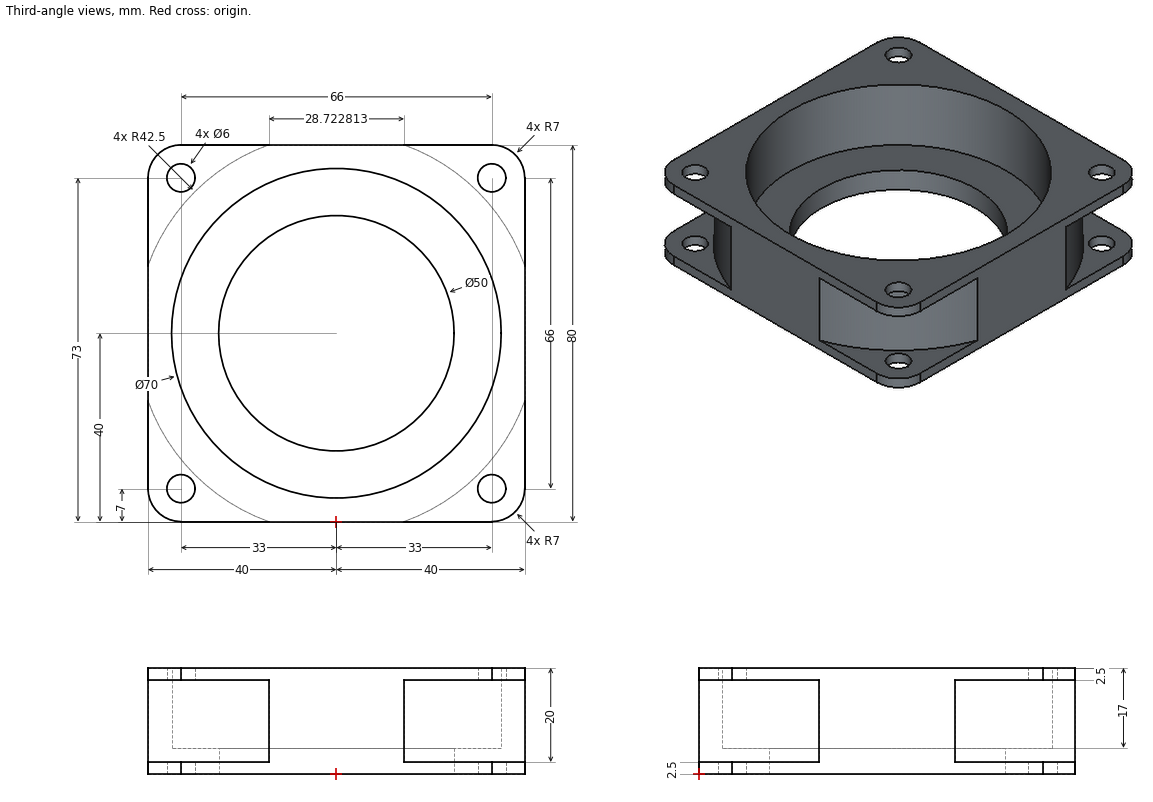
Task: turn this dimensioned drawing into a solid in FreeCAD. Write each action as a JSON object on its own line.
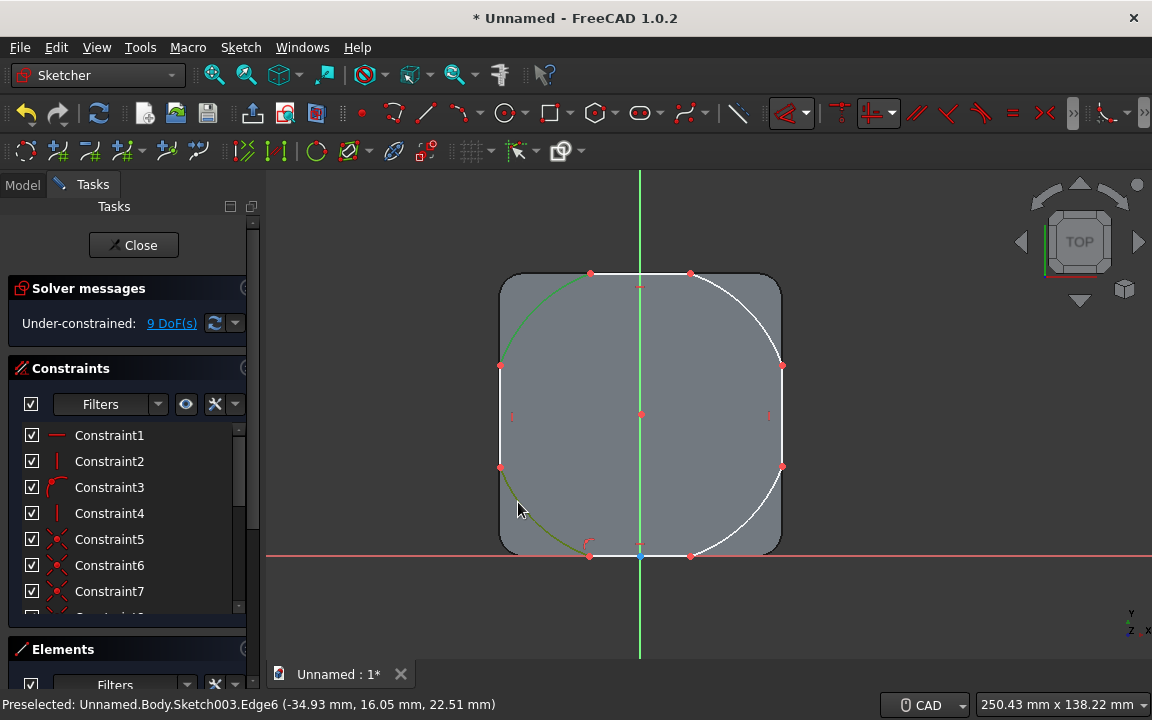
{"action": "left_click", "coordinate": [726, 538]}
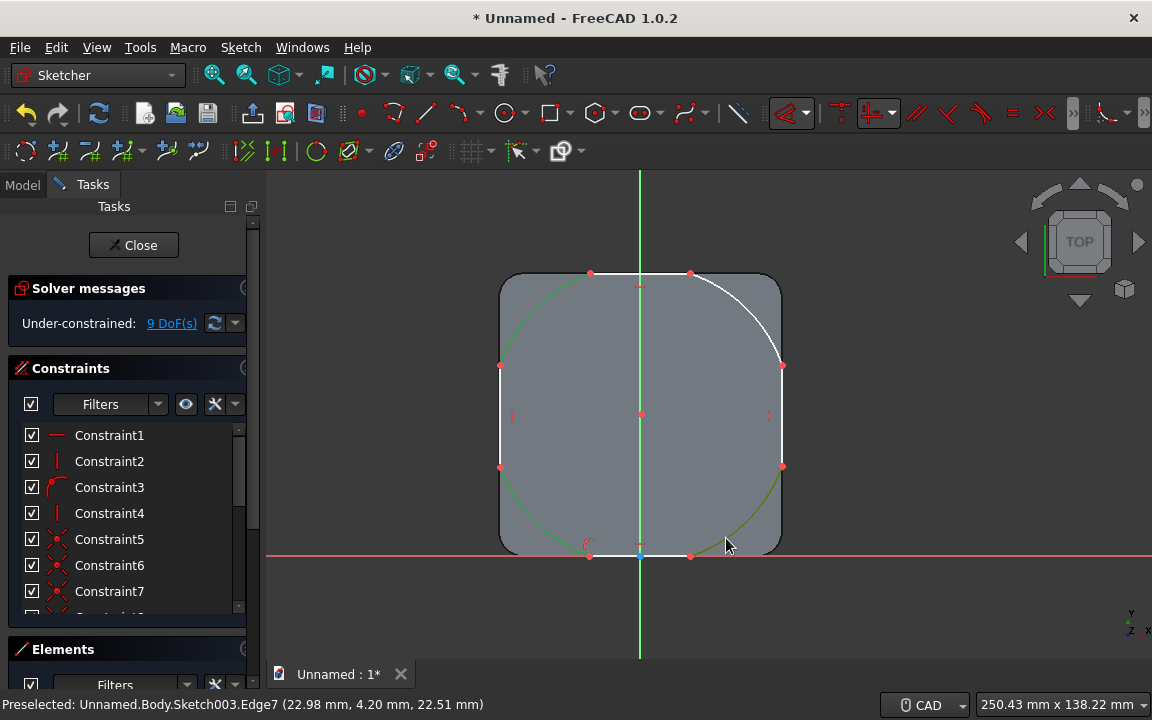
{"action": "left_click", "coordinate": [764, 330]}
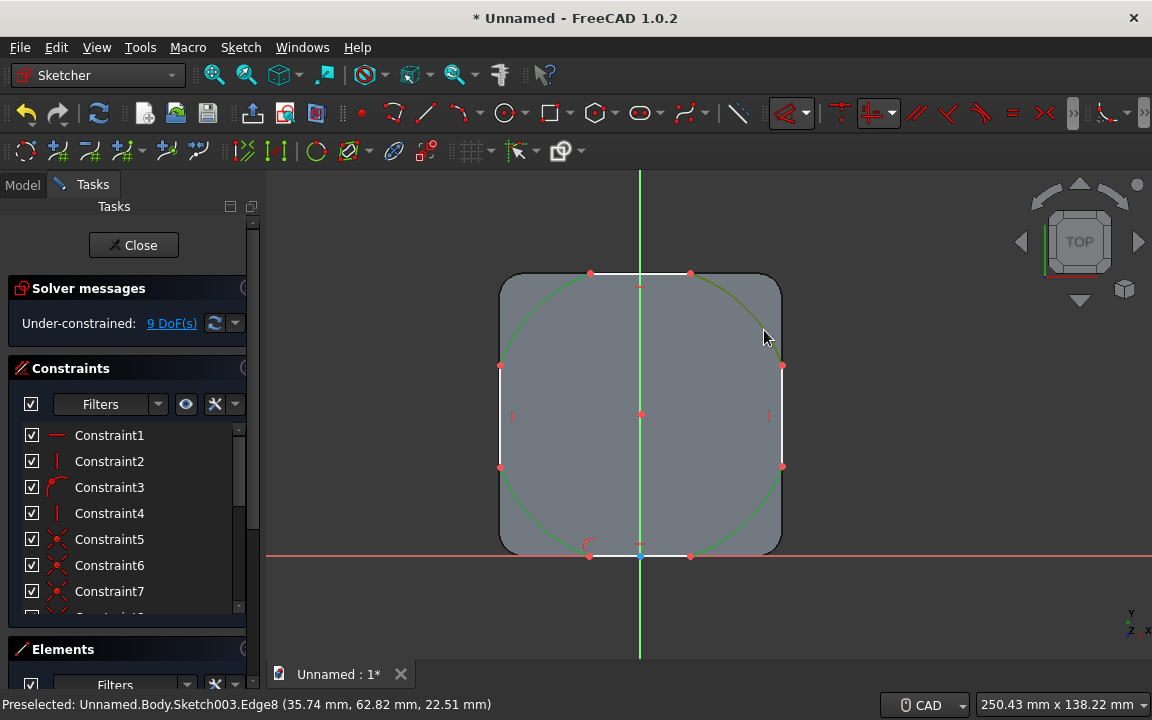
{"action": "left_click", "coordinate": [1014, 114]}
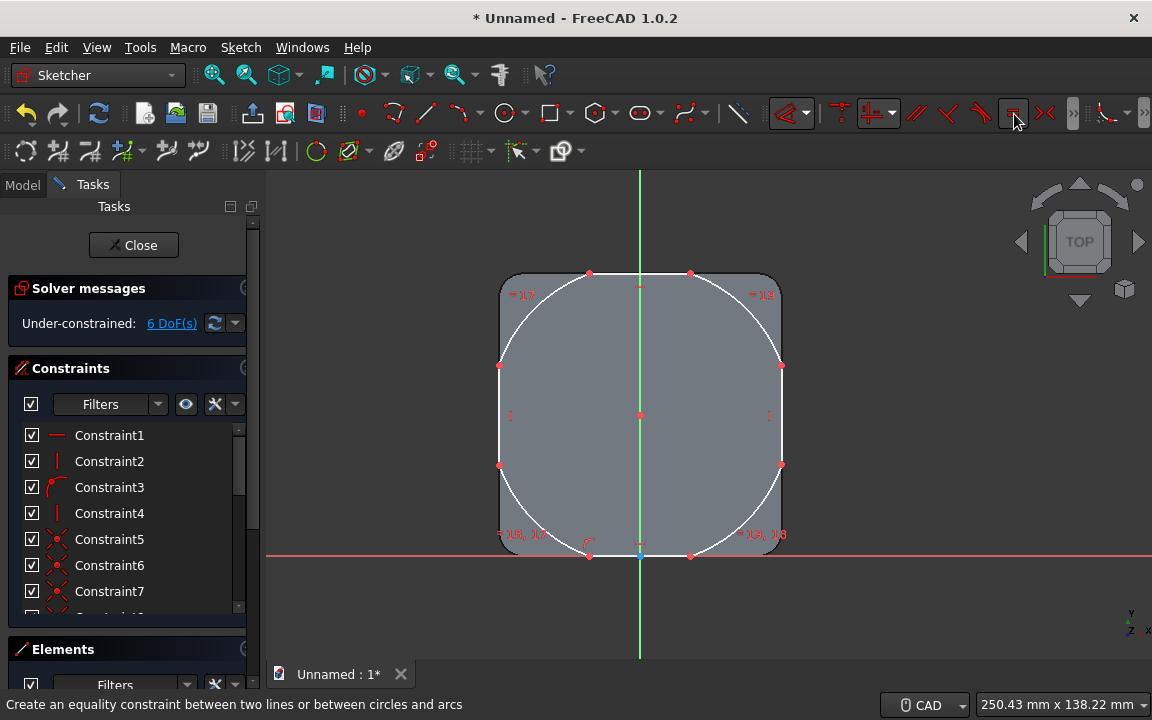
{"action": "left_click", "coordinate": [640, 415]}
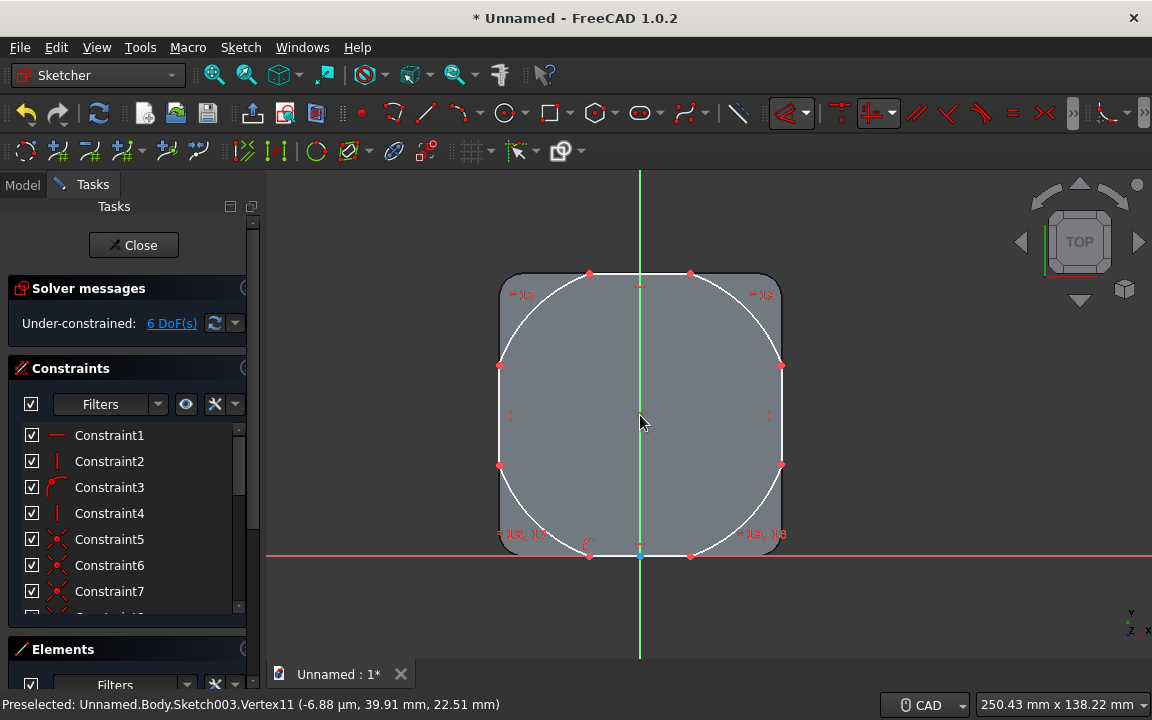
{"action": "left_click", "coordinate": [640, 600]}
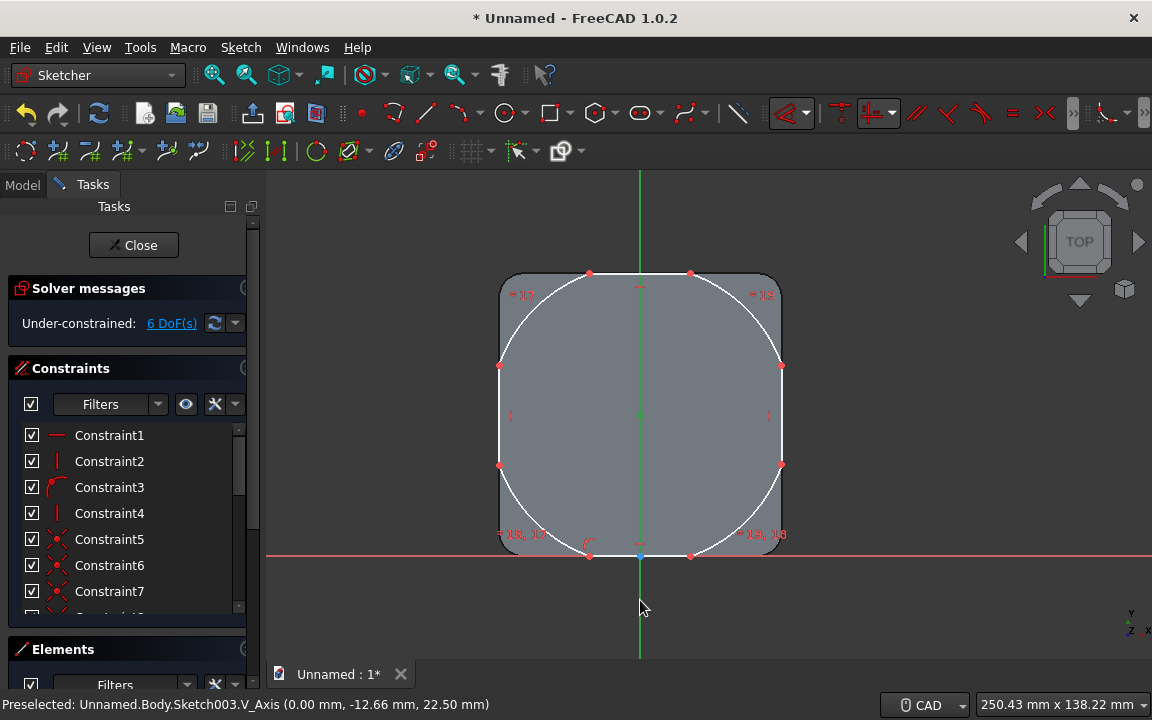
{"action": "left_click", "coordinate": [840, 114]}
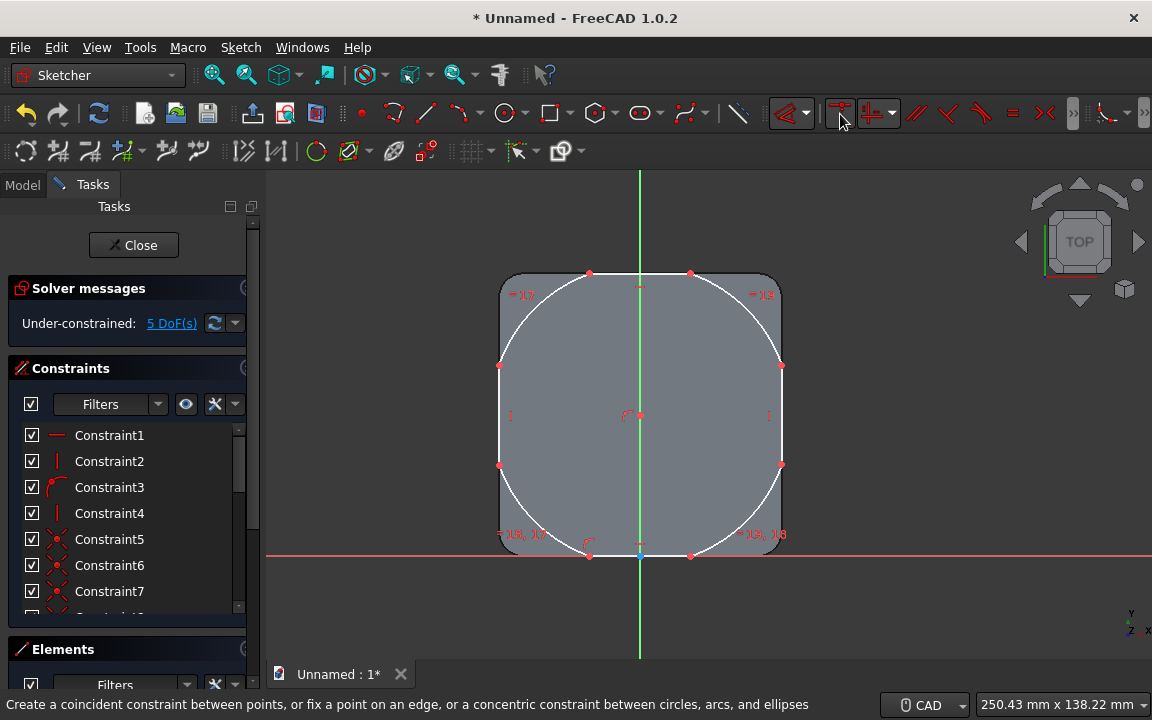
{"action": "key", "text": "d"}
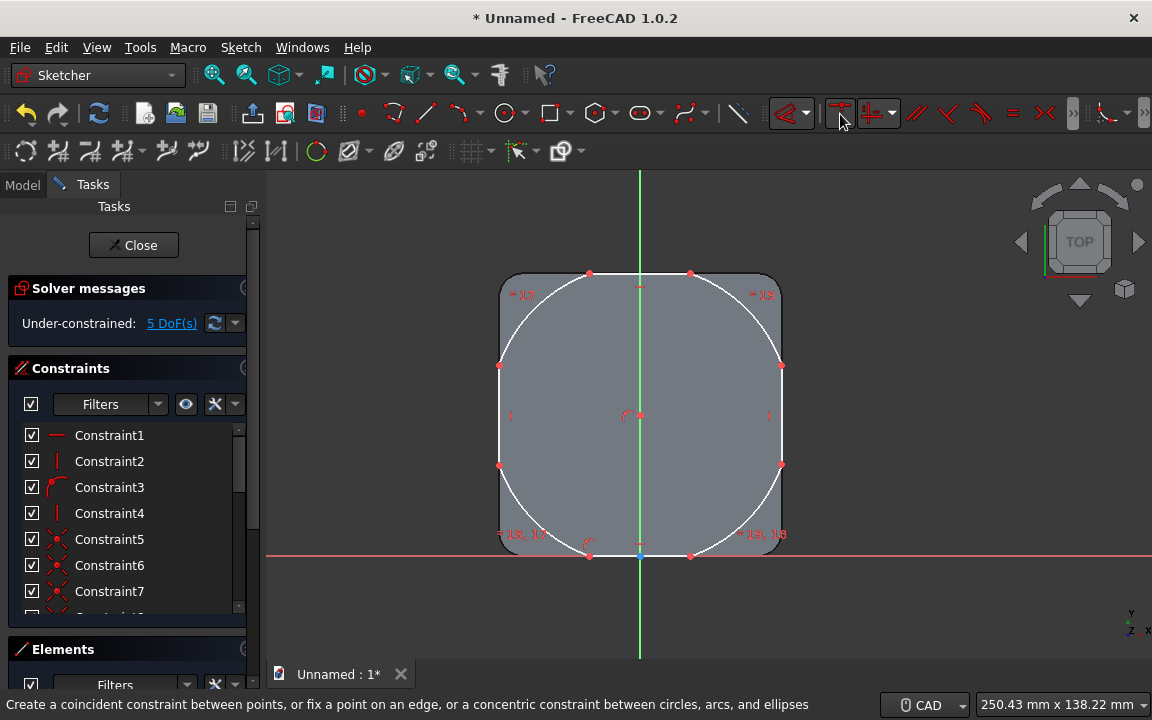
{"action": "left_click", "coordinate": [555, 292]}
{"action": "left_click", "coordinate": [537, 266]}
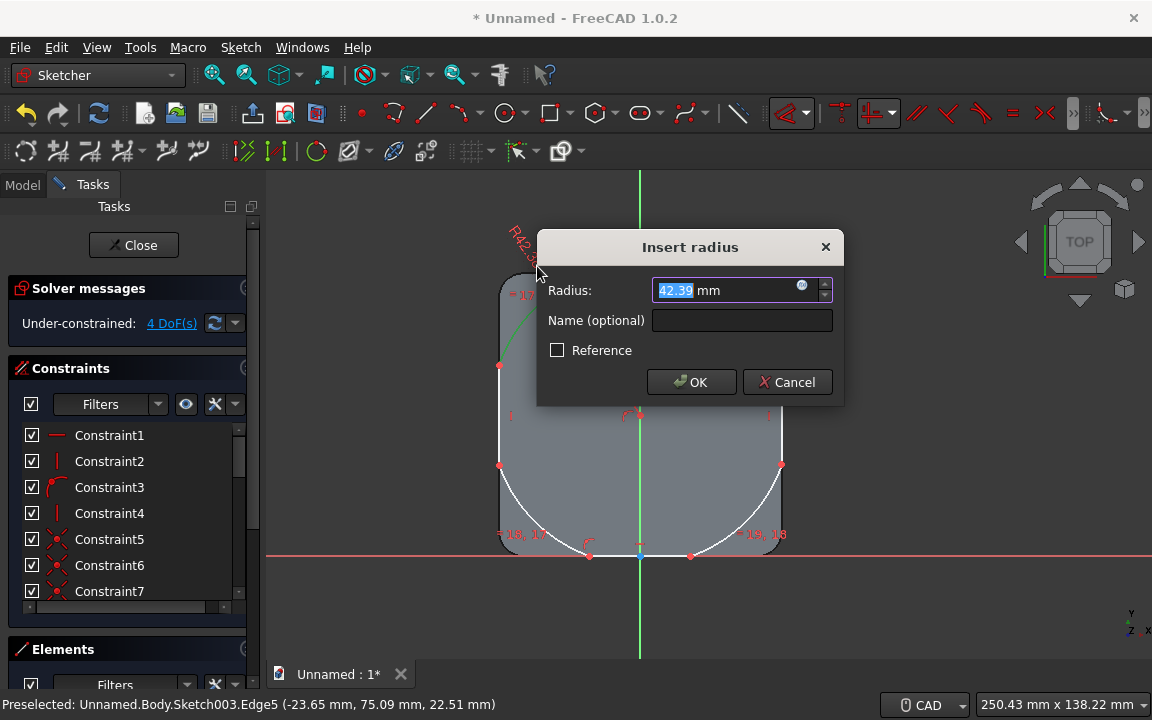
{"action": "type", "text": "42.5"}
{"action": "key", "text": "Return"}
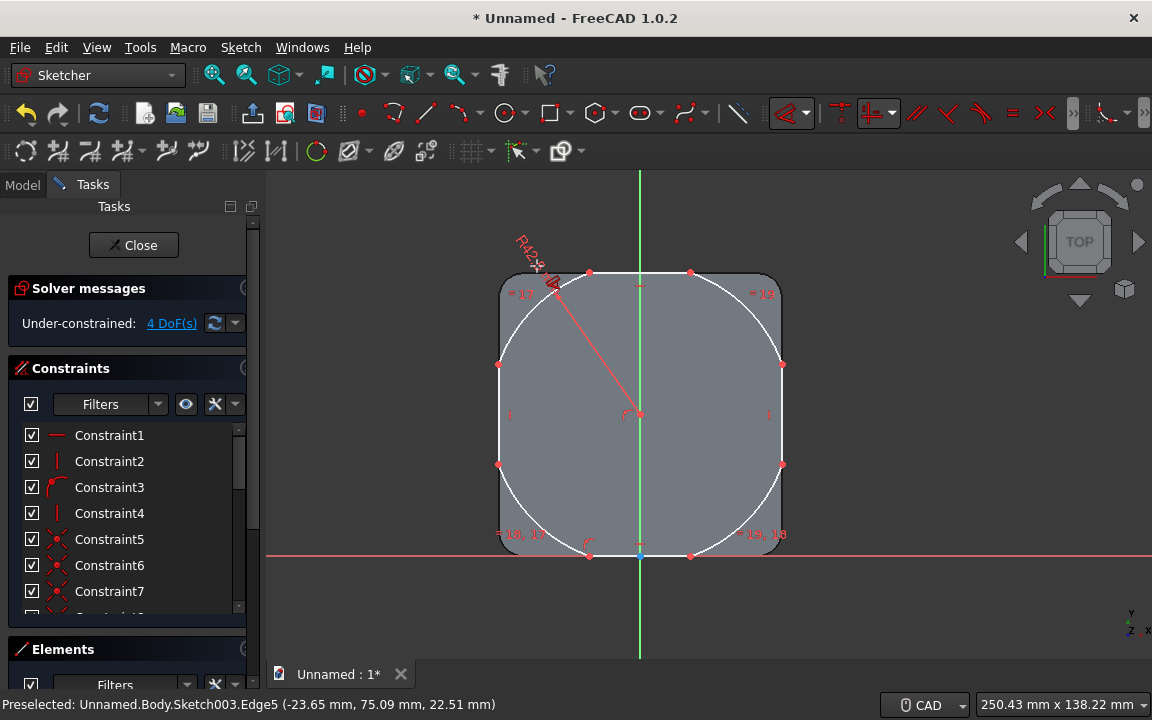
{"action": "left_click", "coordinate": [691, 273]}
{"action": "left_click", "coordinate": [725, 415]}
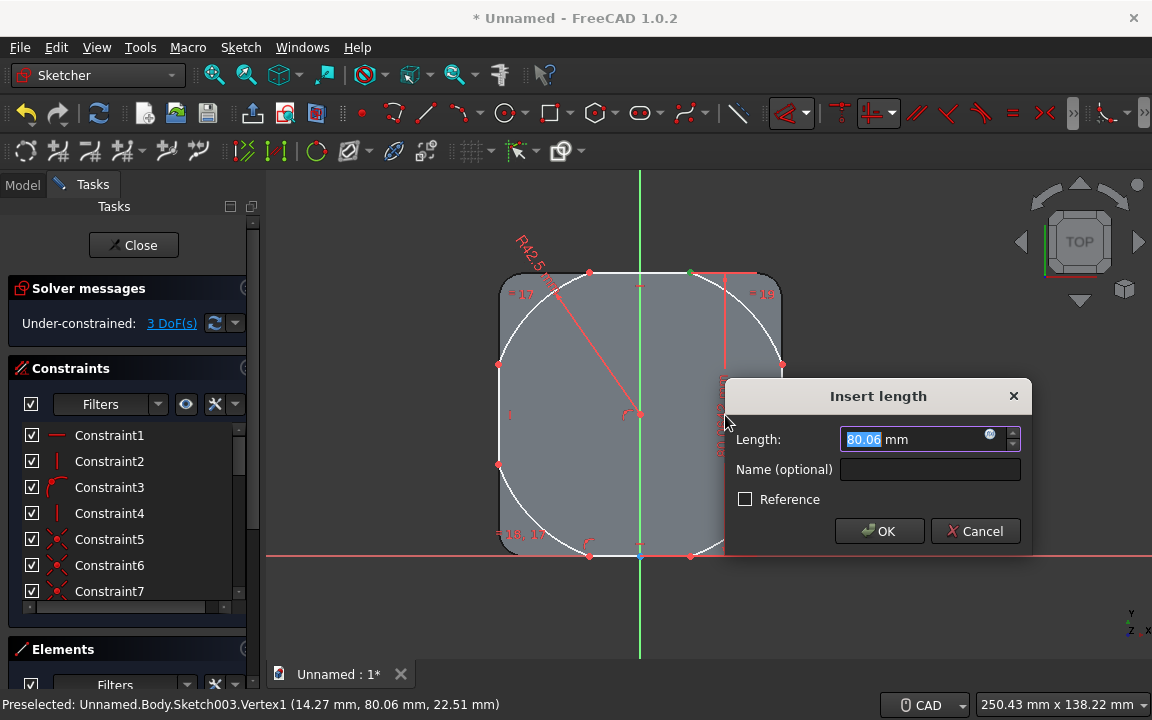
{"action": "type", "text": "80"}
{"action": "key", "text": "Return"}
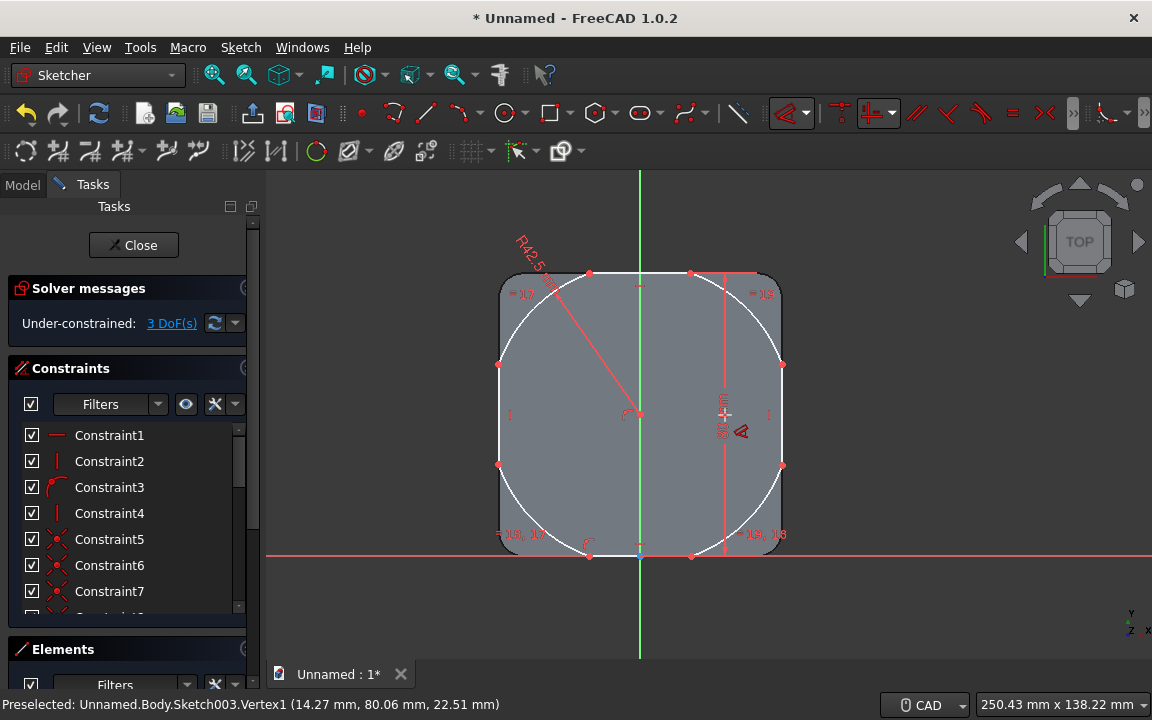
{"action": "left_click", "coordinate": [499, 365]}
{"action": "left_click", "coordinate": [570, 590]}